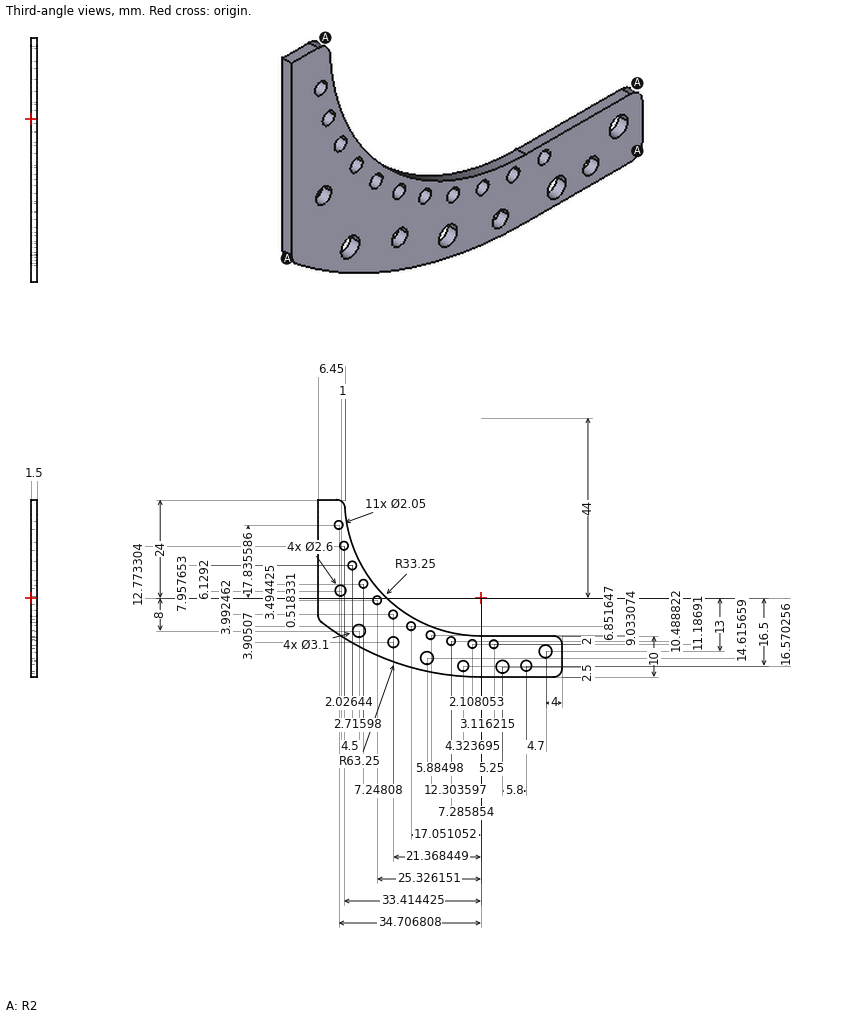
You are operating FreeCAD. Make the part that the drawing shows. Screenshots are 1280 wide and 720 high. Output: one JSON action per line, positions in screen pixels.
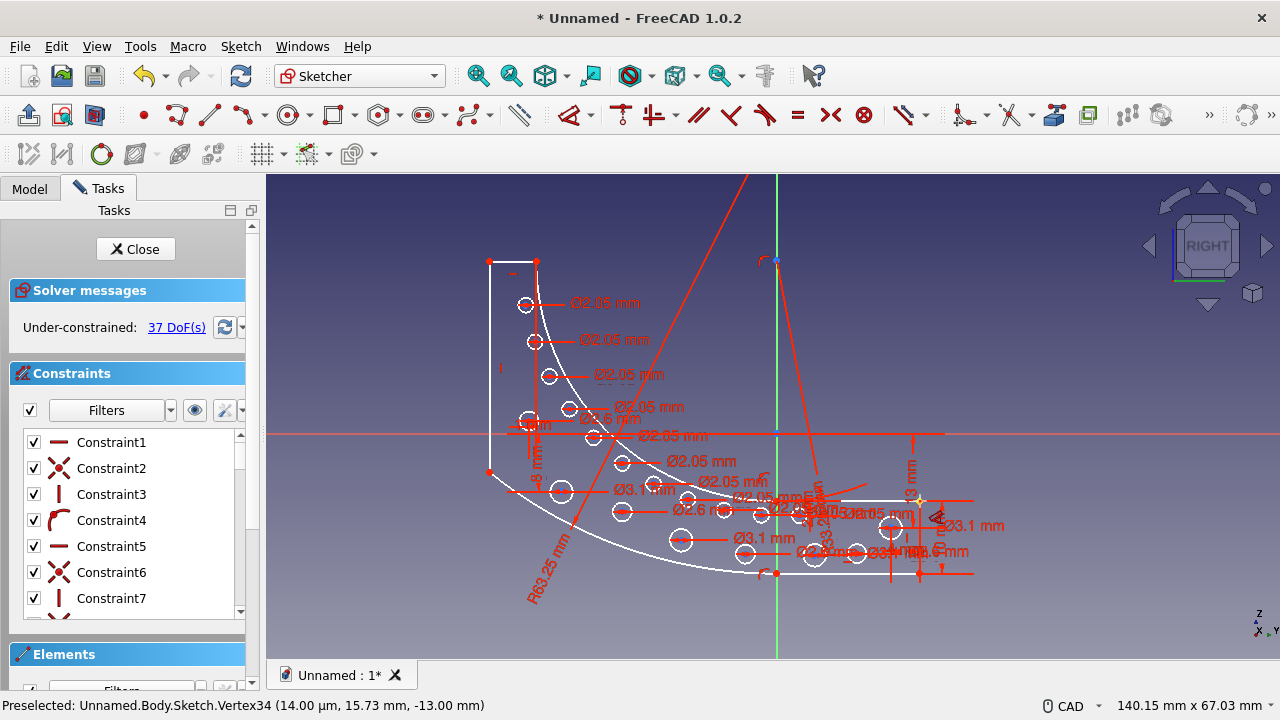
{"action": "left_click", "coordinate": [536, 262]}
{"action": "left_click", "coordinate": [811, 348]}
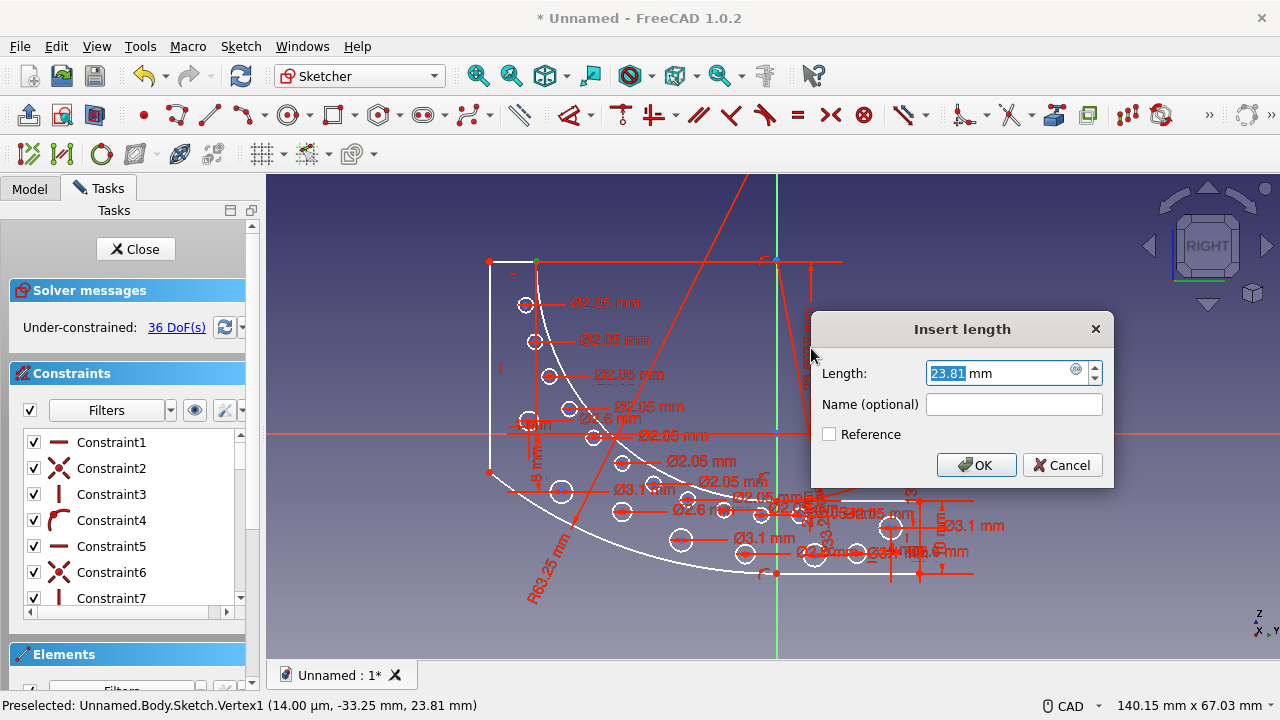
{"action": "type", "text": "24"}
{"action": "key", "text": "Return"}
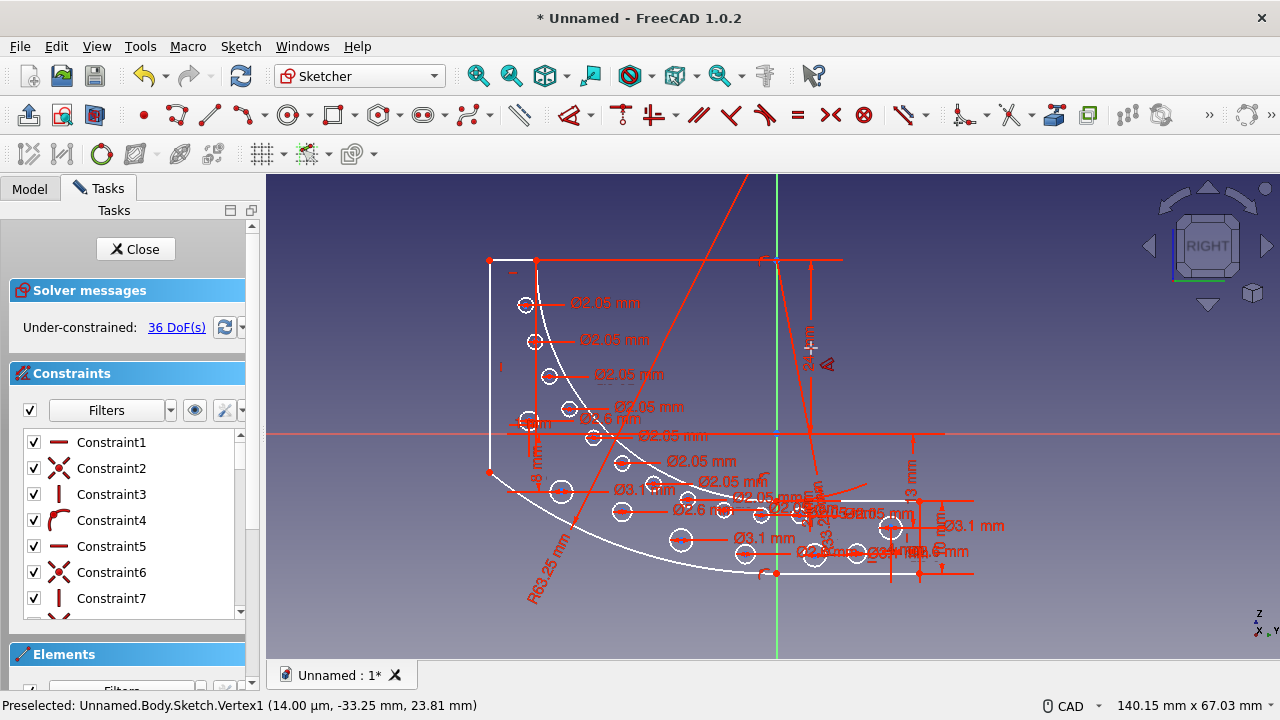
{"action": "scroll", "coordinate": [704, 563], "scroll_direction": "down", "scroll_amount": 2}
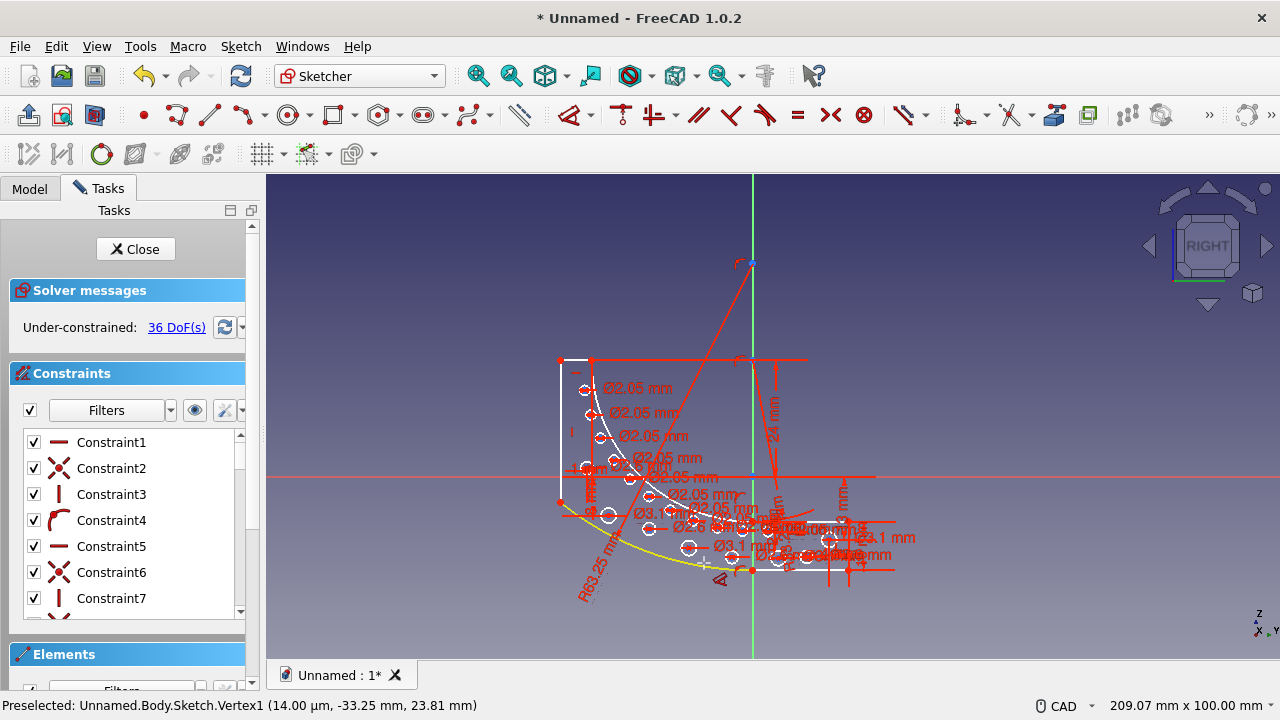
{"action": "left_click", "coordinate": [753, 264]}
{"action": "left_click", "coordinate": [787, 370]}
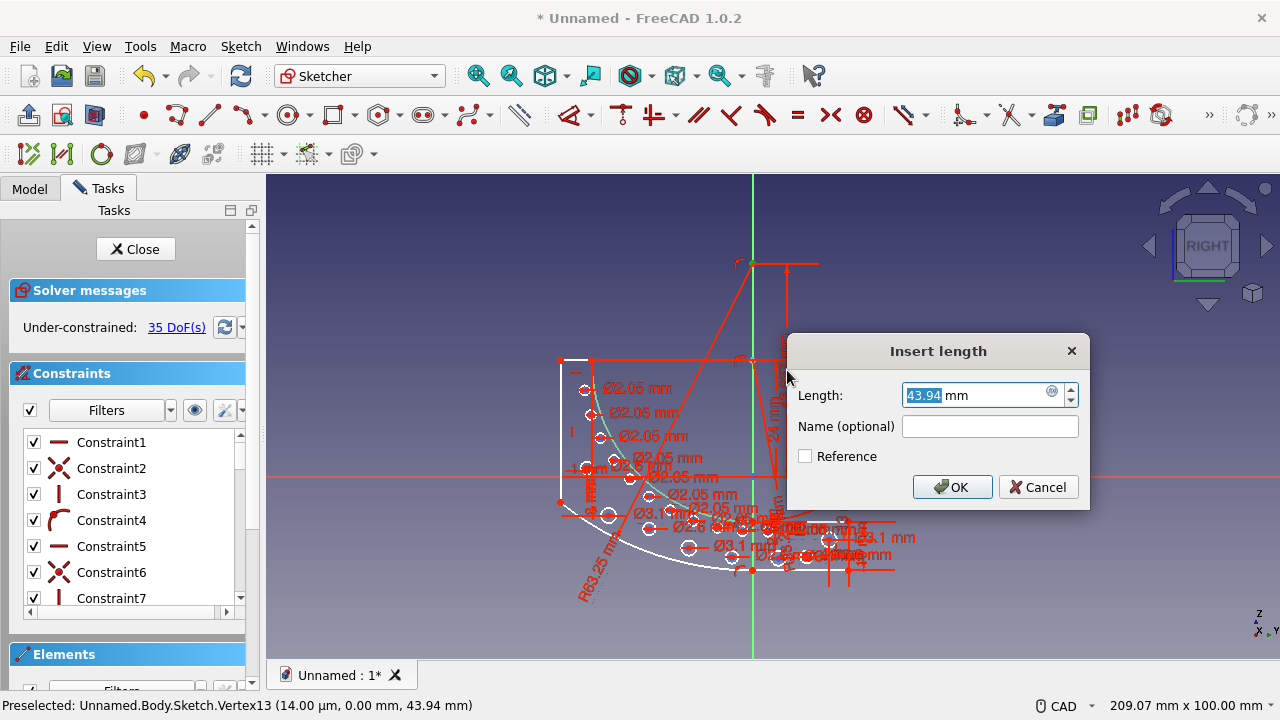
{"action": "type", "text": "44"}
{"action": "key", "text": "Return"}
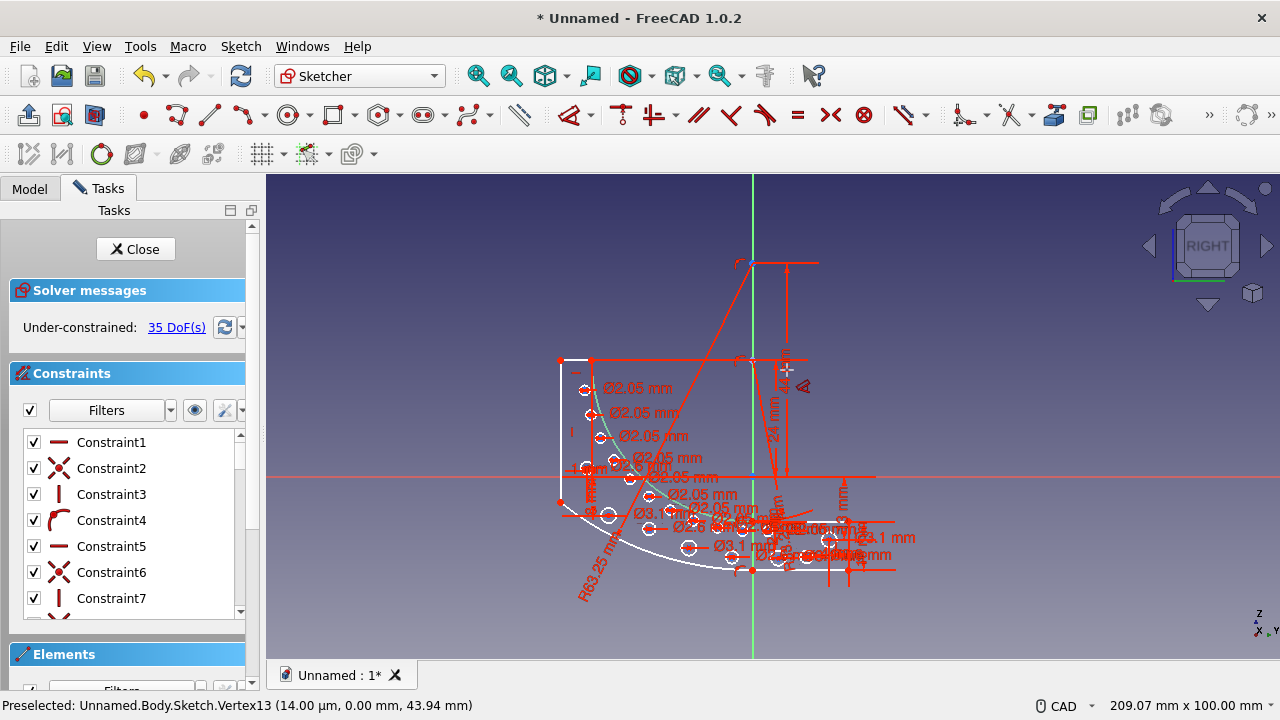
{"action": "scroll", "coordinate": [582, 360], "scroll_direction": "up", "scroll_amount": 2}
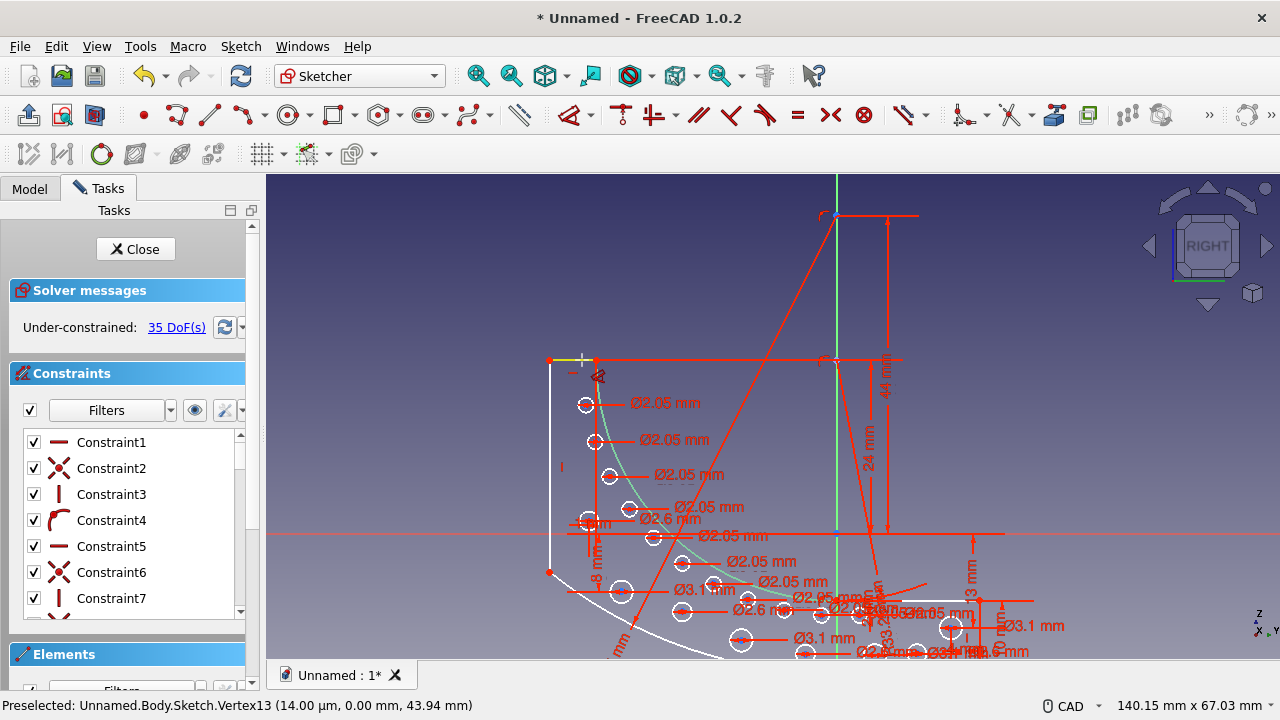
{"action": "left_click", "coordinate": [582, 360]}
{"action": "left_click", "coordinate": [573, 326]}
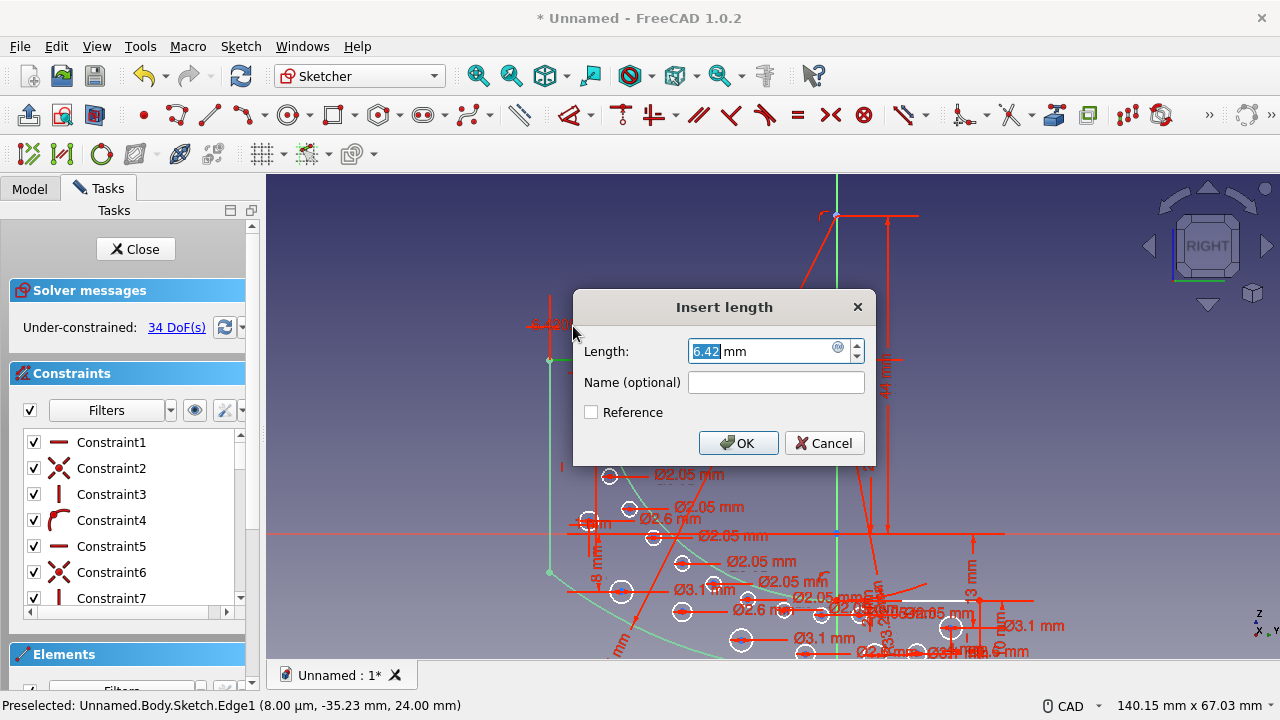
{"action": "type", "text": "6.45"}
{"action": "key", "text": "Return"}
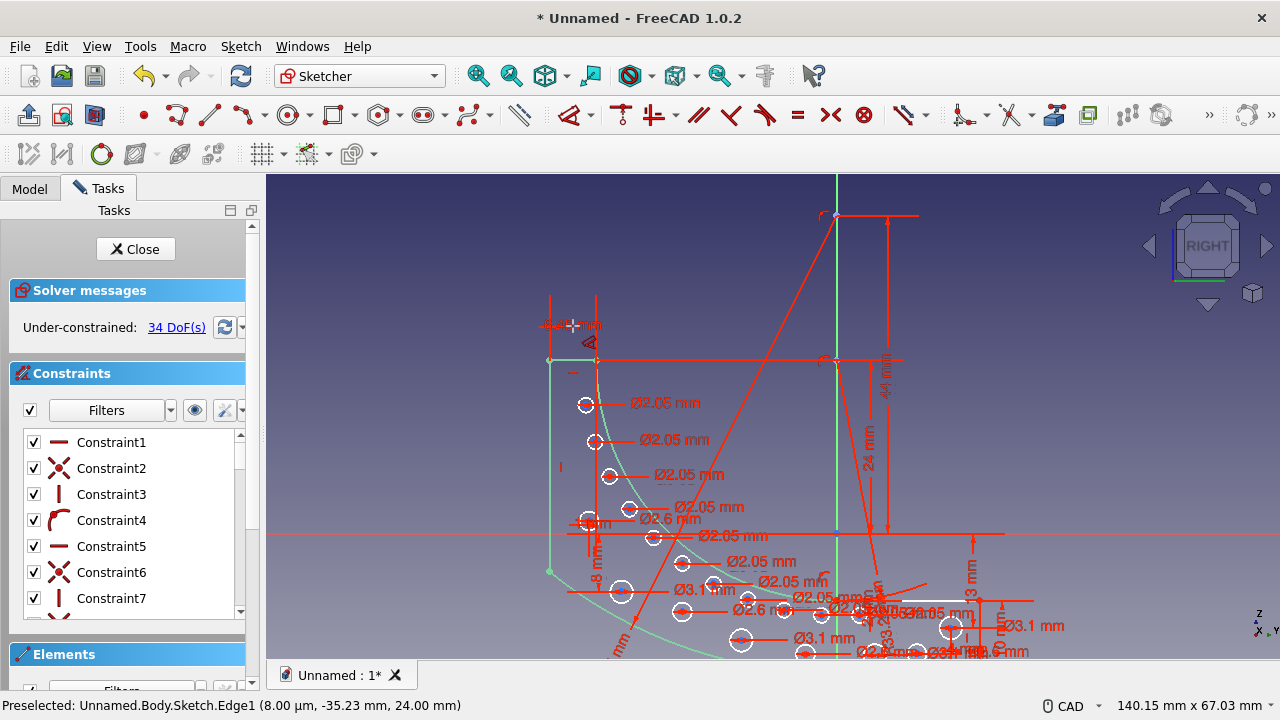
{"action": "scroll", "coordinate": [432, 202], "scroll_direction": "down", "scroll_amount": 1}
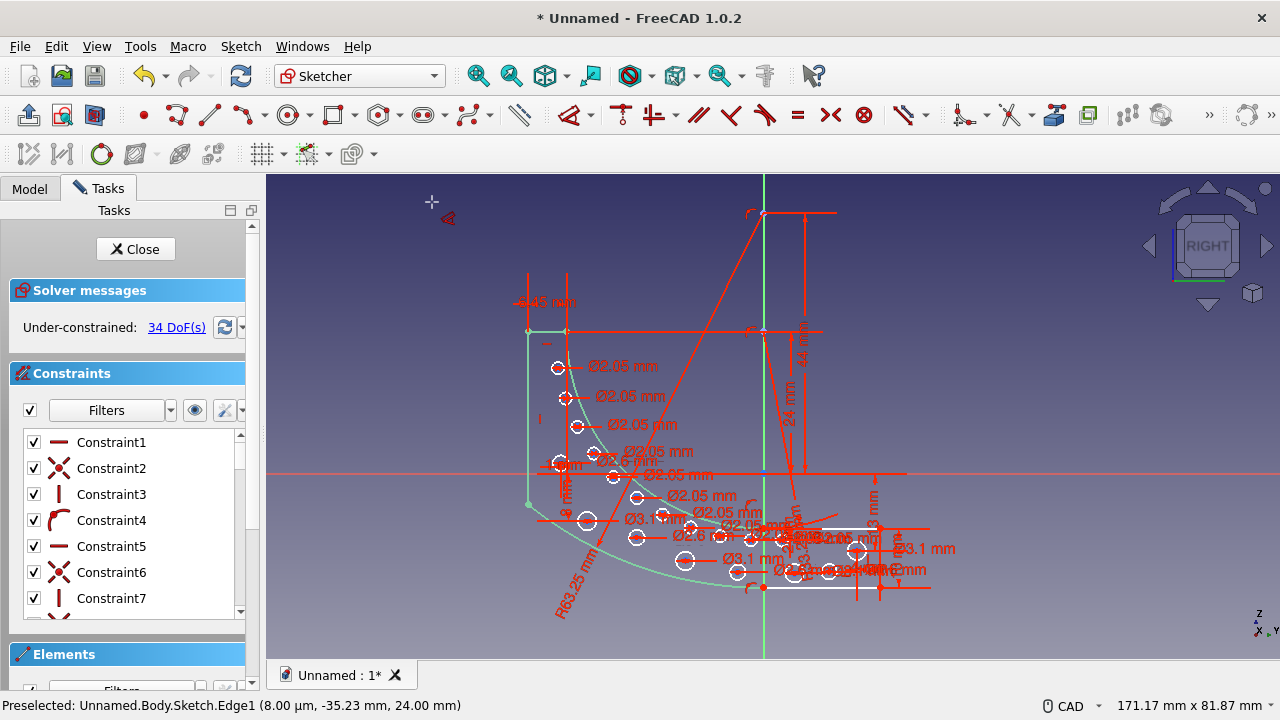
{"action": "scroll", "coordinate": [795, 573], "scroll_direction": "up", "scroll_amount": 2}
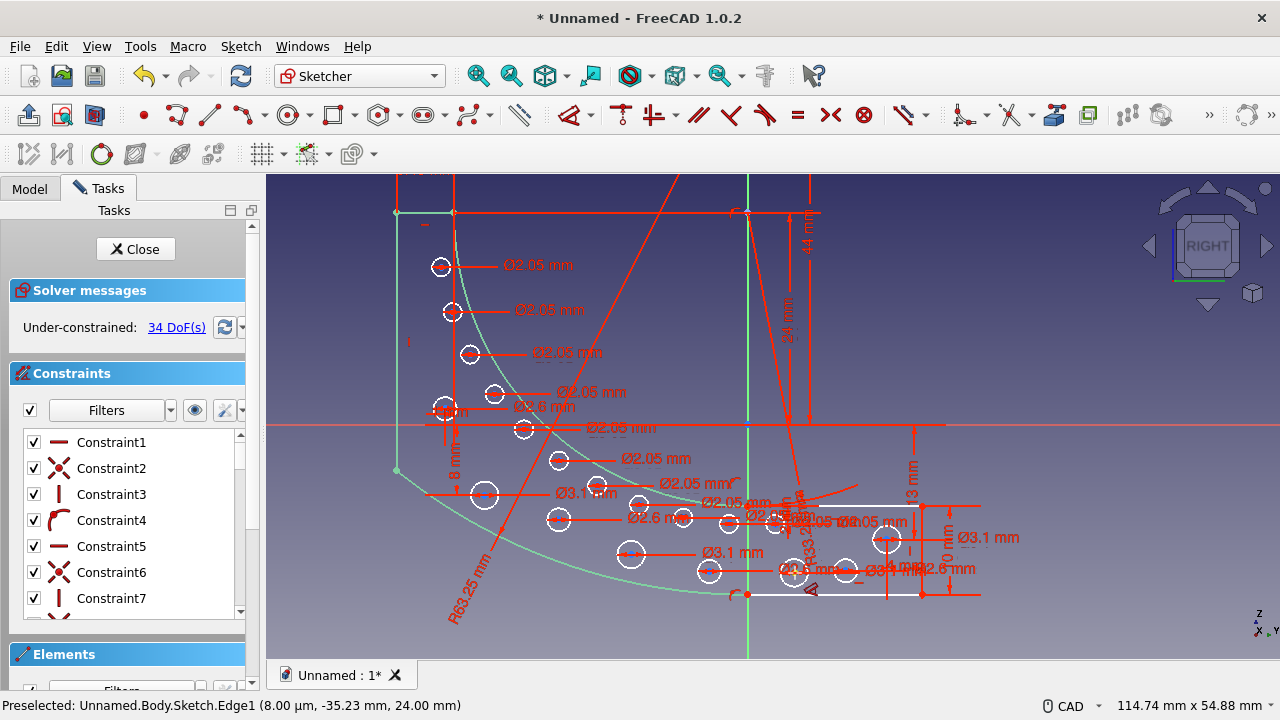
{"action": "left_click", "coordinate": [794, 573]}
{"action": "left_click", "coordinate": [771, 391]}